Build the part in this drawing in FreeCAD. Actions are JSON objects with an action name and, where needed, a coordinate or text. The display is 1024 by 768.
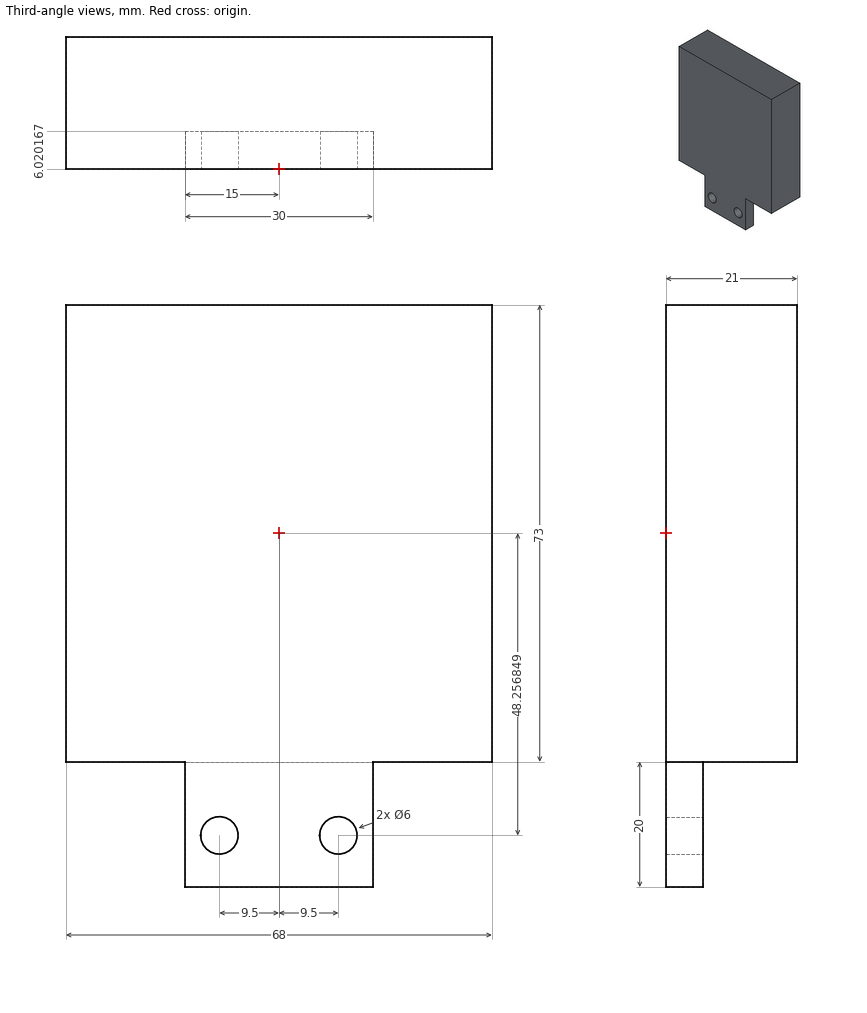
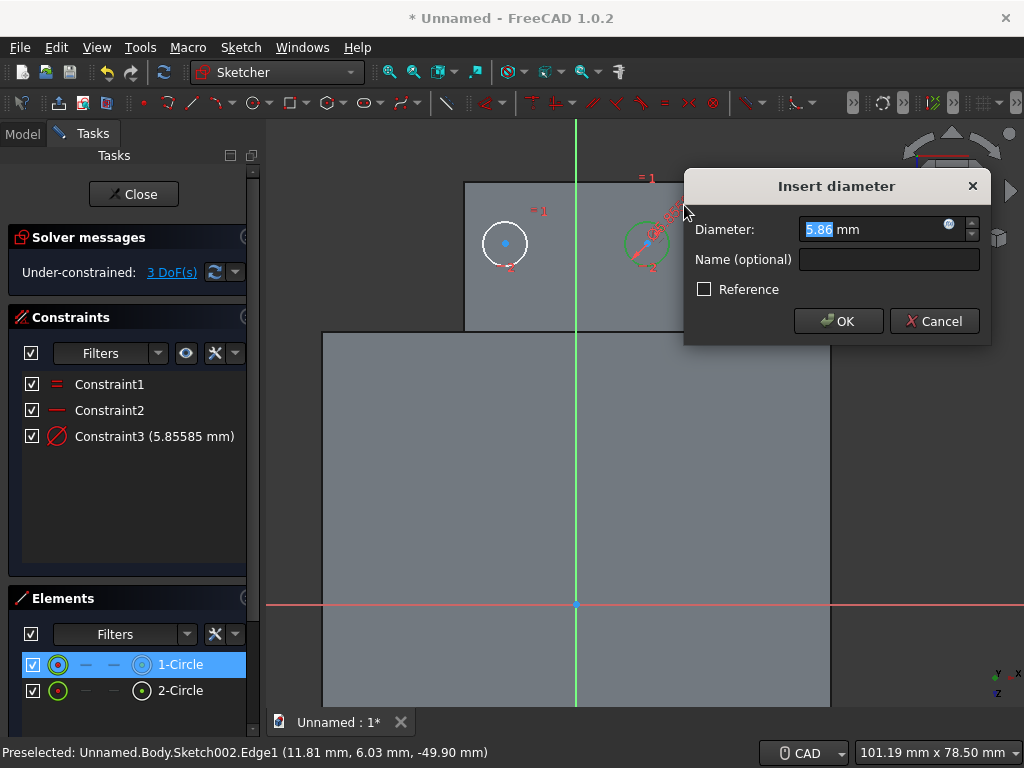
{"action": "type", "text": "6"}
{"action": "key", "text": "Return"}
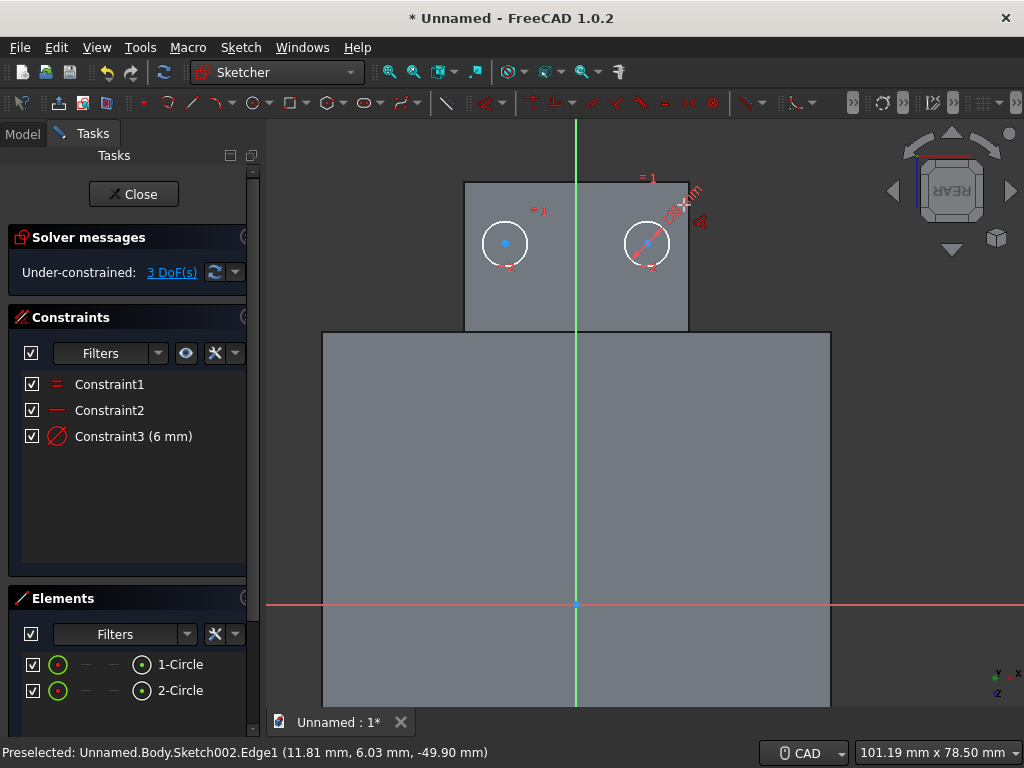
{"action": "left_click", "coordinate": [647, 244]}
{"action": "left_click", "coordinate": [612, 639]}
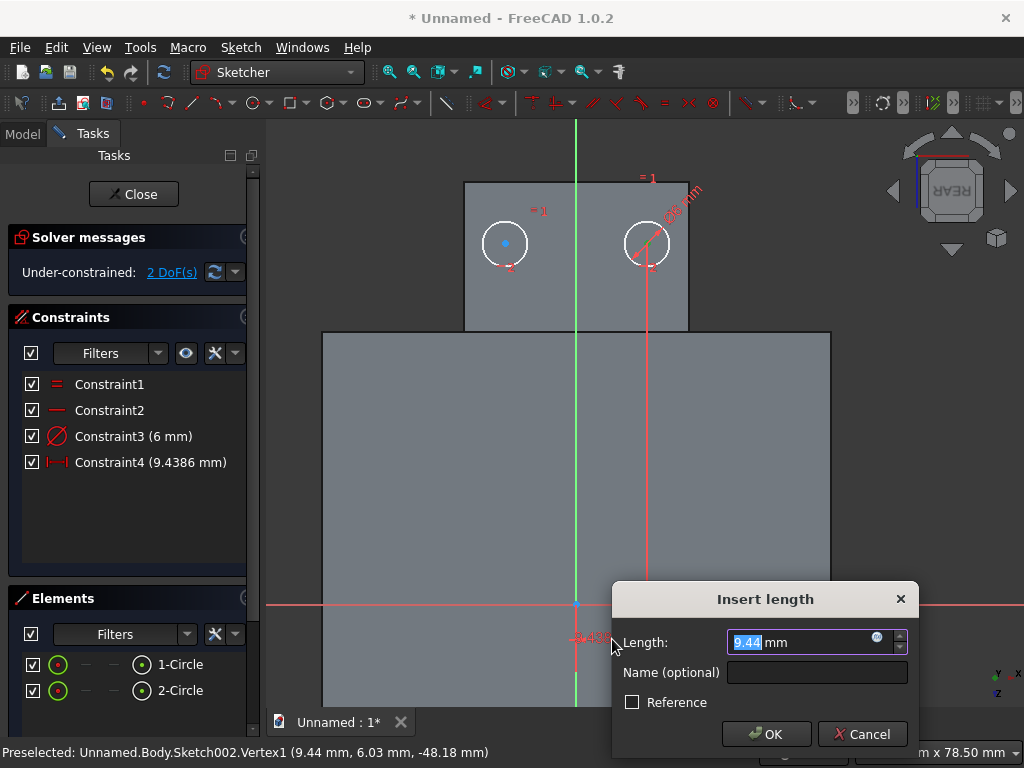
{"action": "type", "text": "9.5"}
{"action": "key", "text": "Return"}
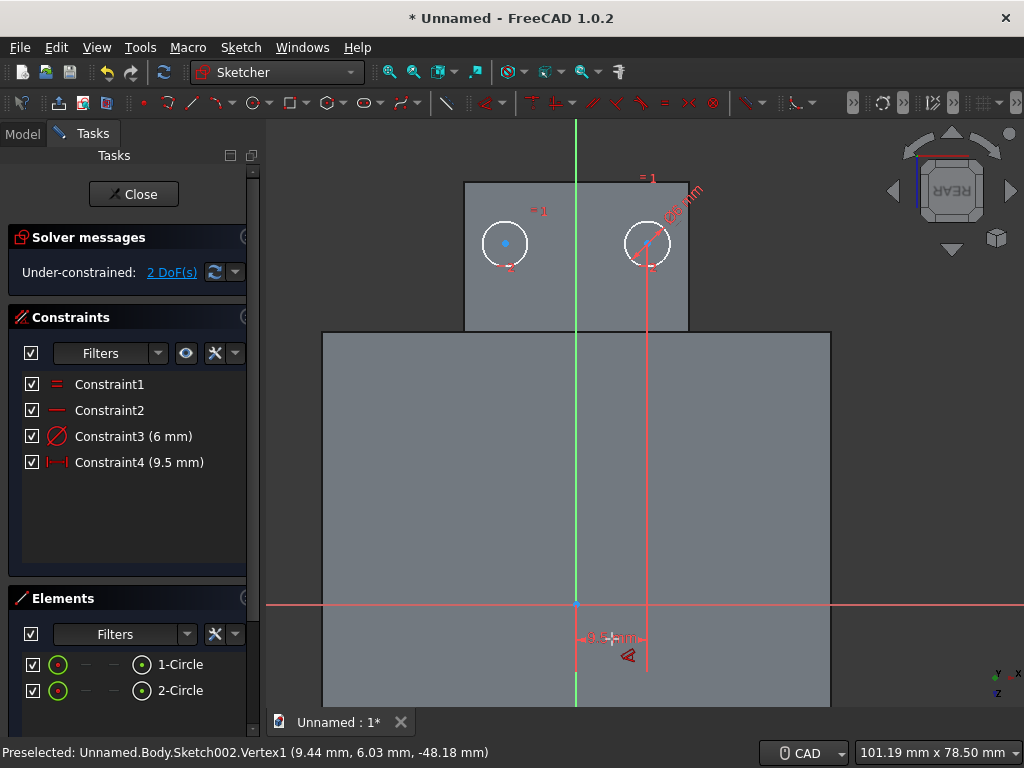
{"action": "left_click", "coordinate": [505, 244]}
{"action": "left_click", "coordinate": [541, 639]}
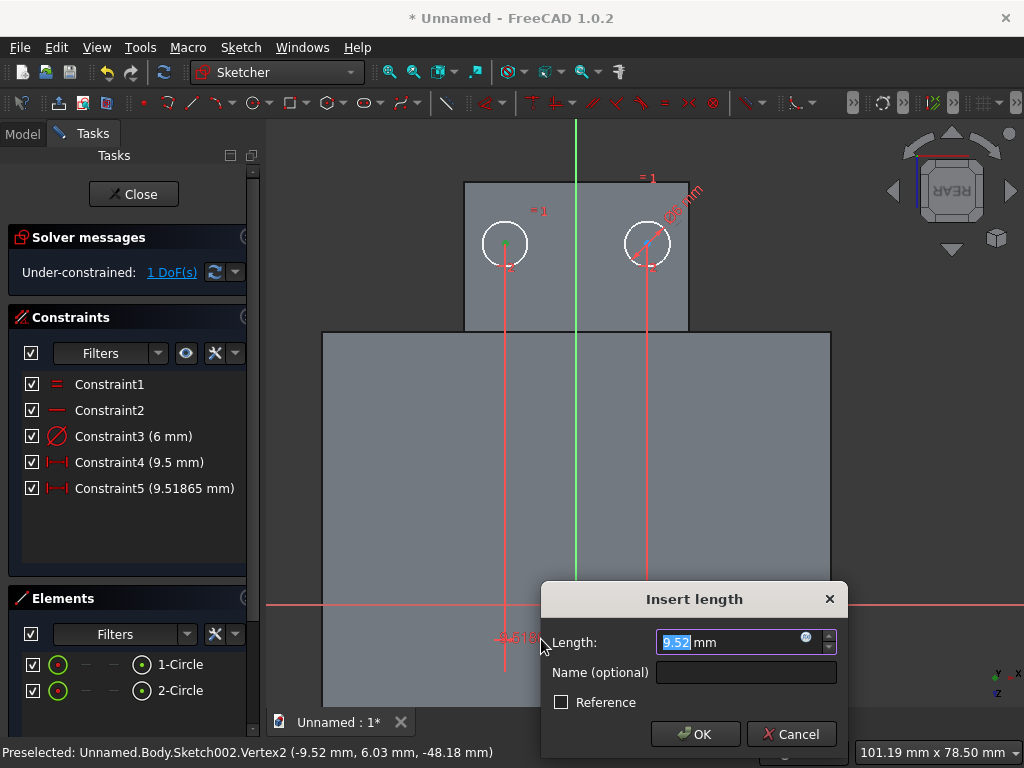
{"action": "type", "text": "9.5"}
{"action": "key", "text": "Return"}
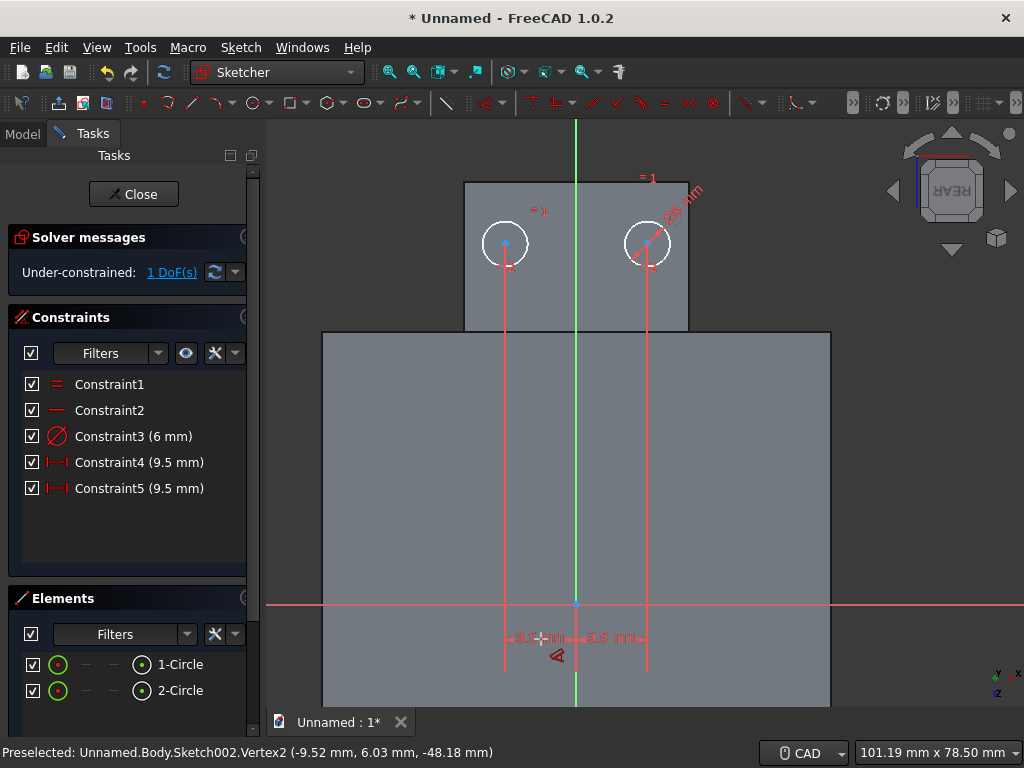
{"action": "left_click", "coordinate": [647, 244]}
{"action": "left_click", "coordinate": [681, 424]}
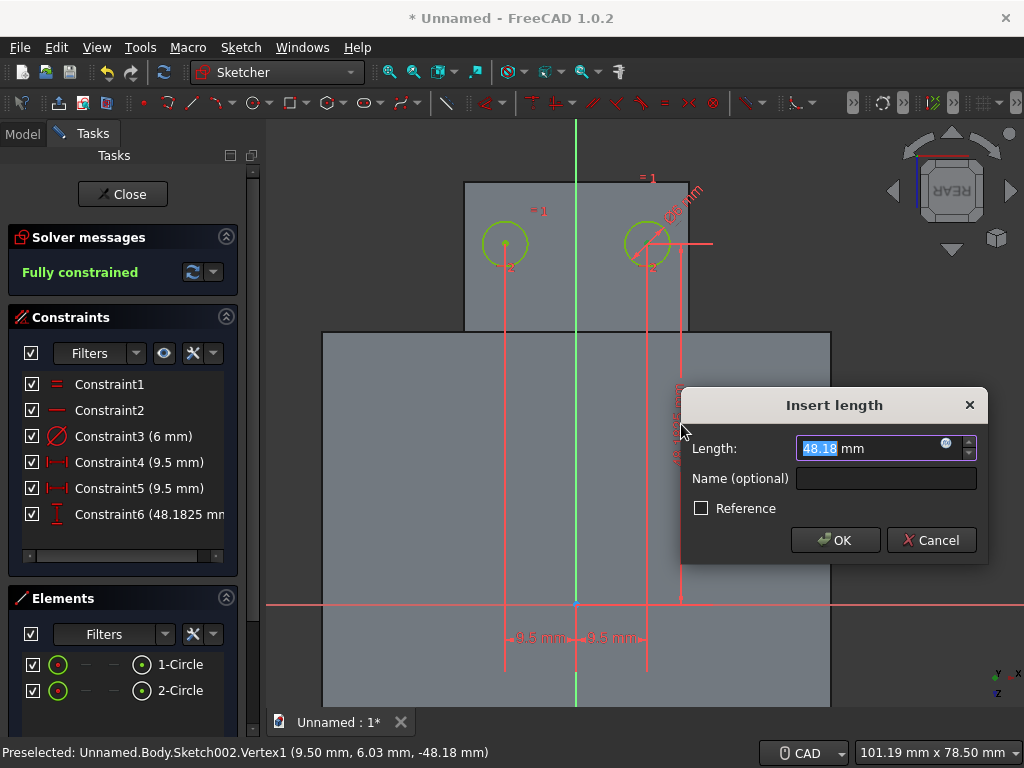
{"action": "type", "text": "48.256849"}
{"action": "key", "text": "Return"}
{"action": "key", "text": "Escape"}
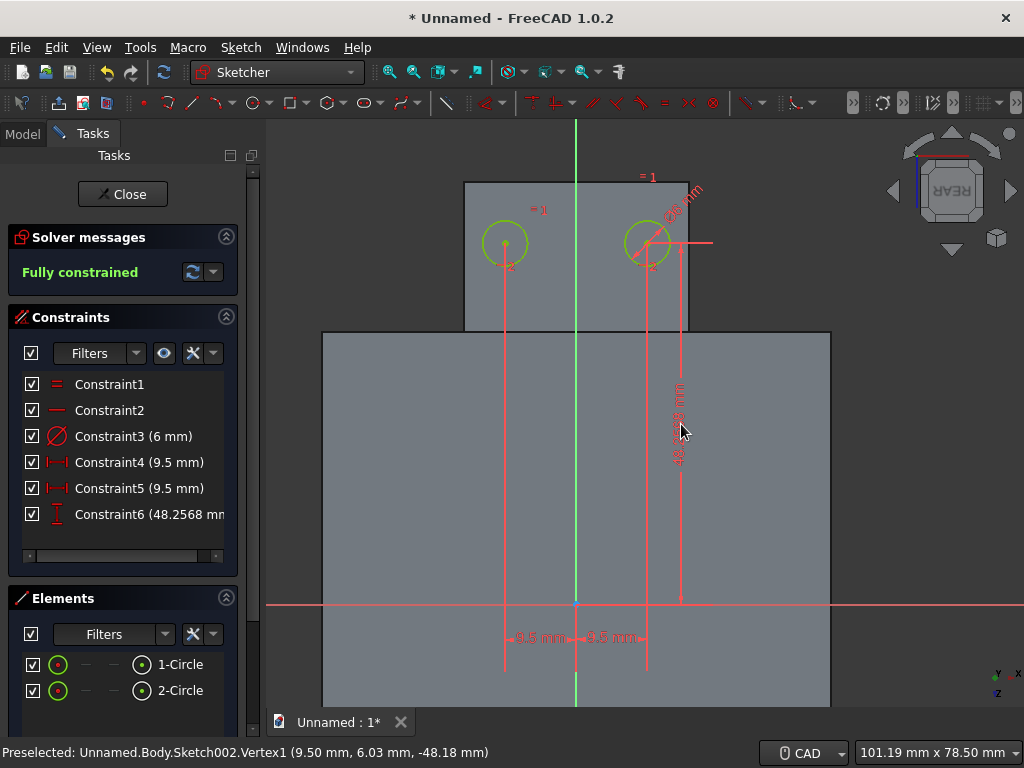
{"action": "left_click", "coordinate": [123, 194]}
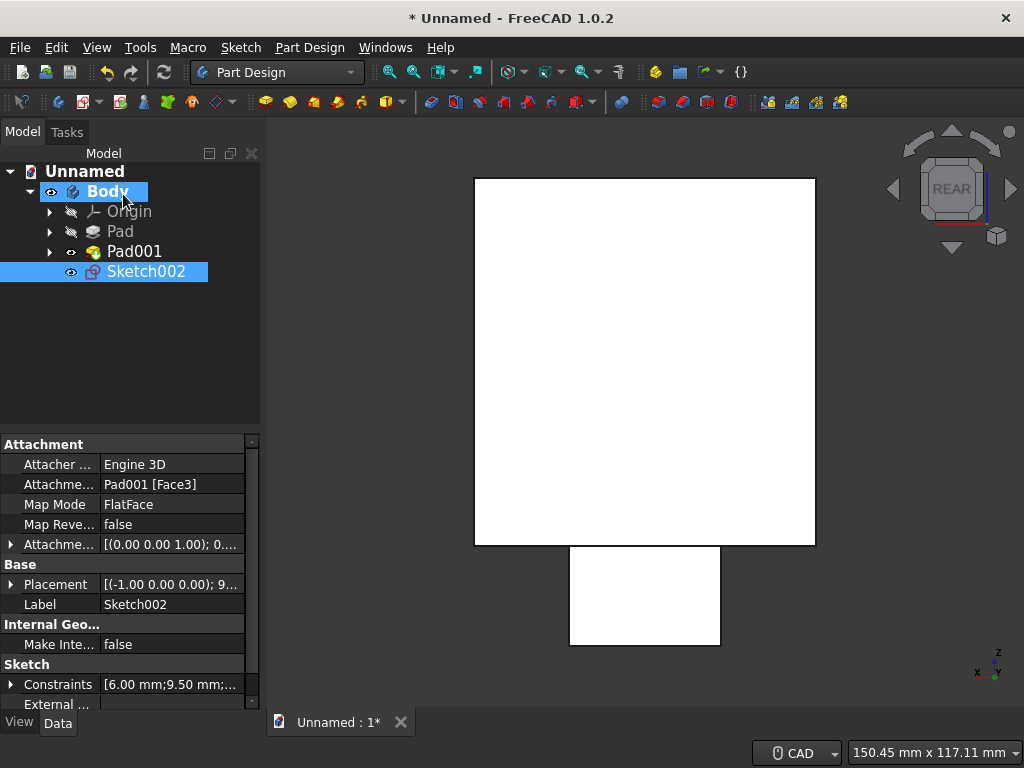
{"action": "left_click", "coordinate": [432, 102]}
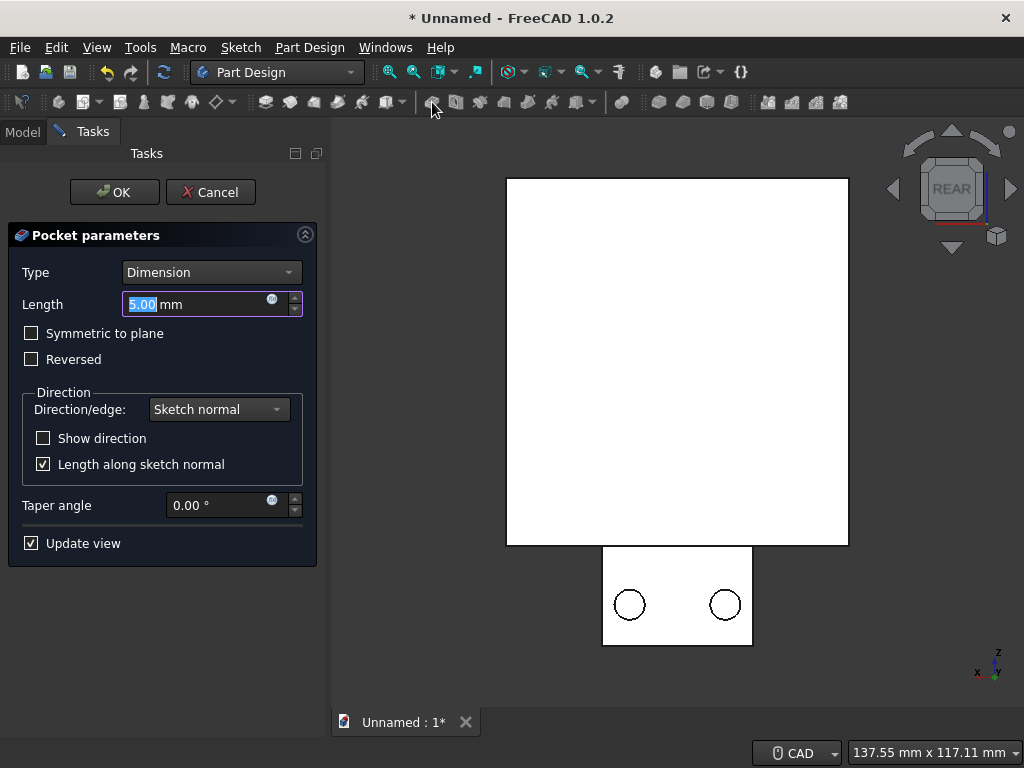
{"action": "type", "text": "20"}
{"action": "key", "text": "Tab"}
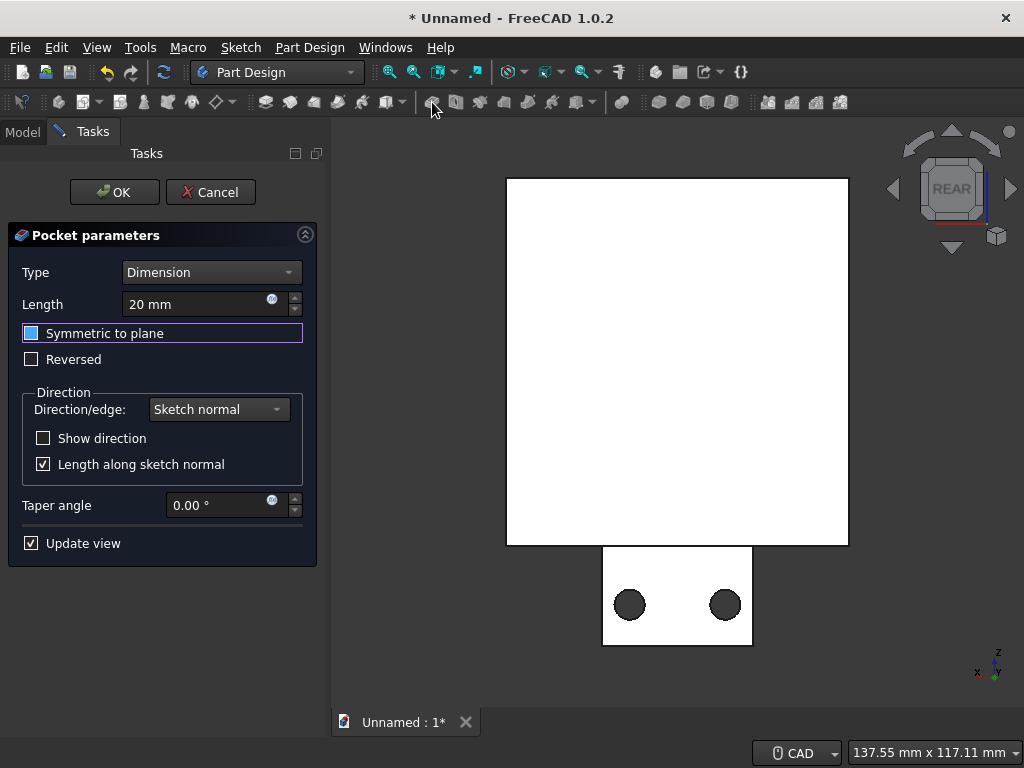
{"action": "left_click", "coordinate": [115, 192]}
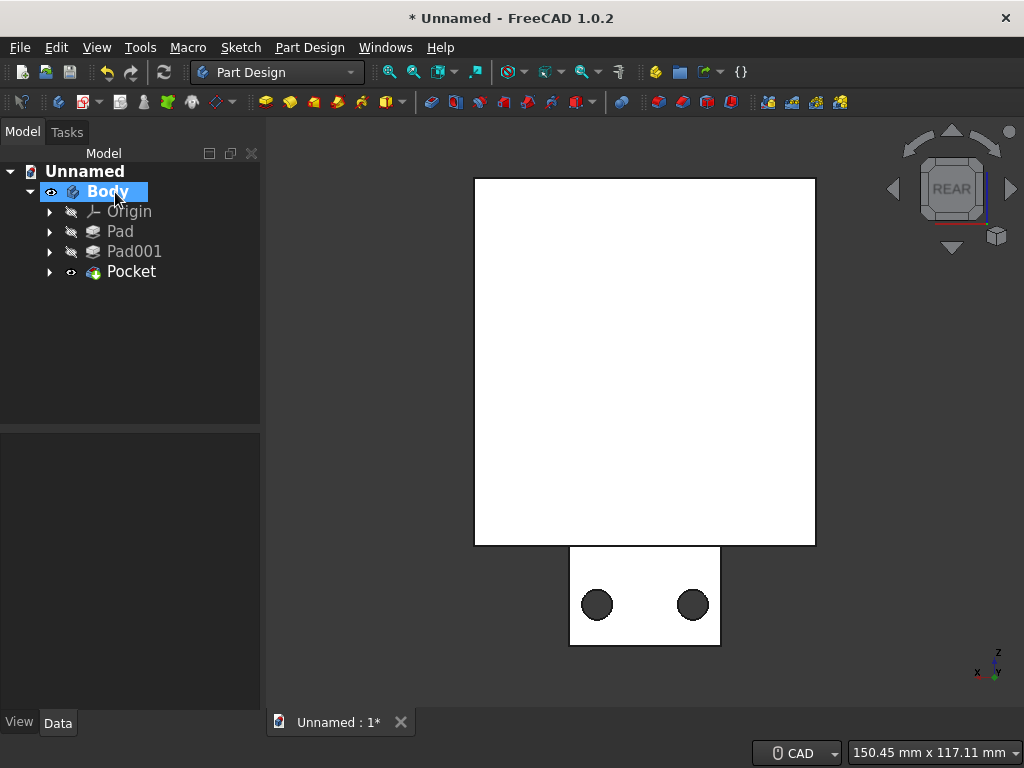
{"action": "key", "text": "0"}